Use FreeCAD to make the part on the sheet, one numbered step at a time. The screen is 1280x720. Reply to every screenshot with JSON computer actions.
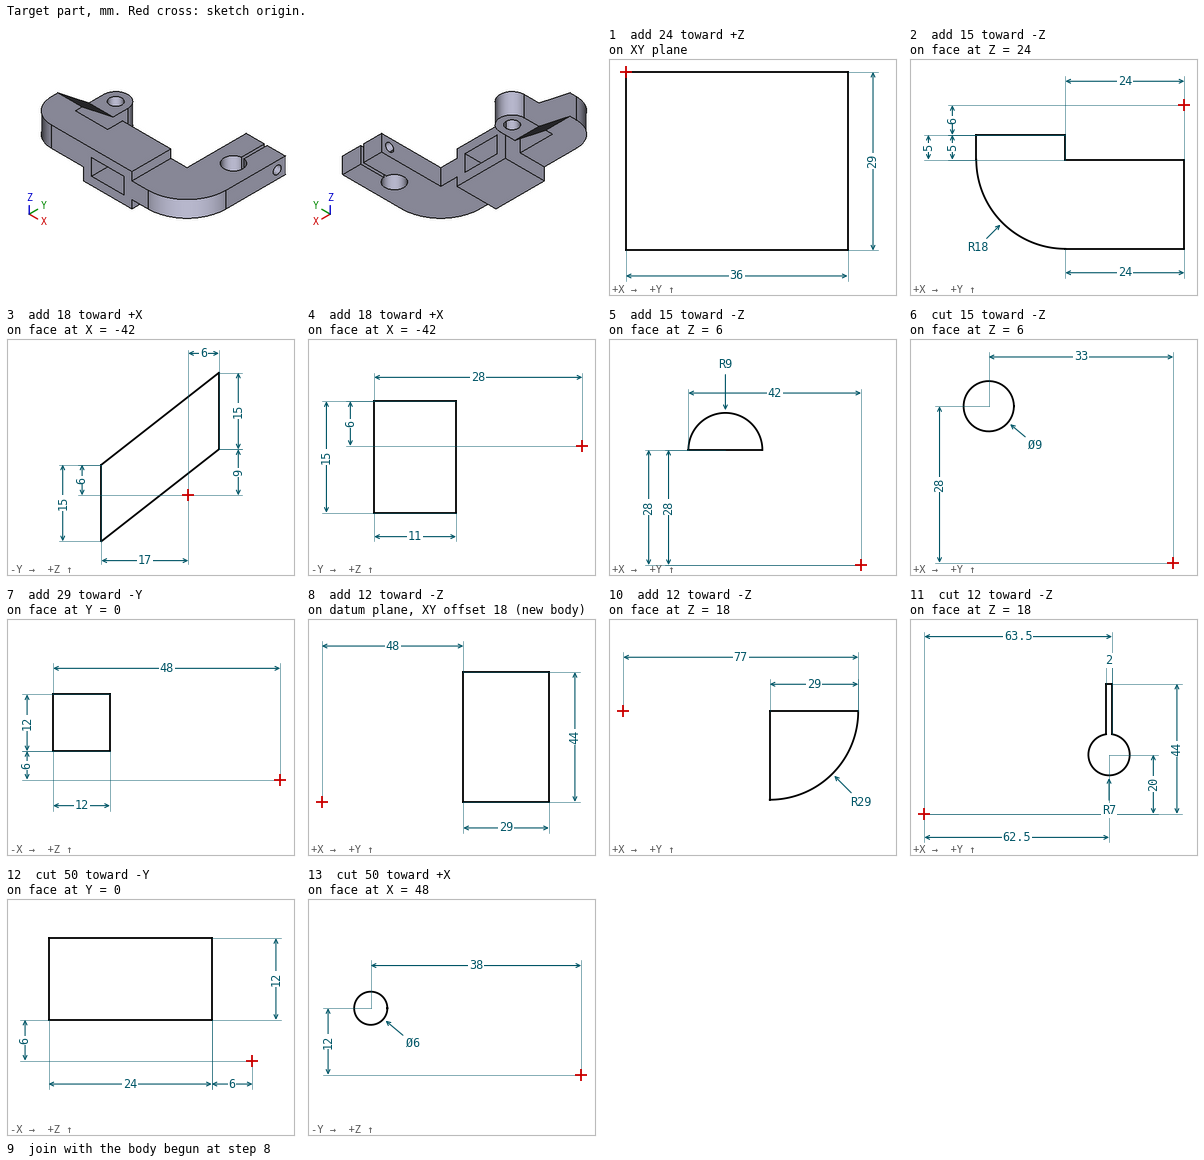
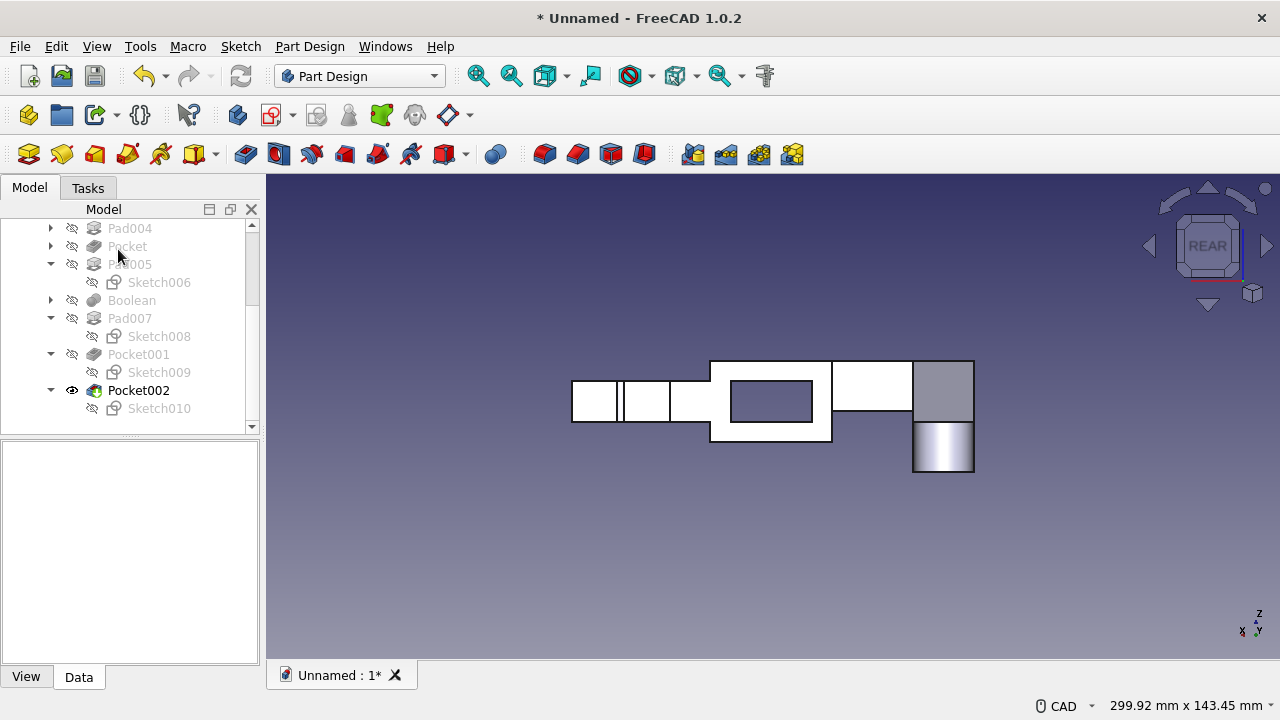
{"action": "left_click", "coordinate": [479, 76]}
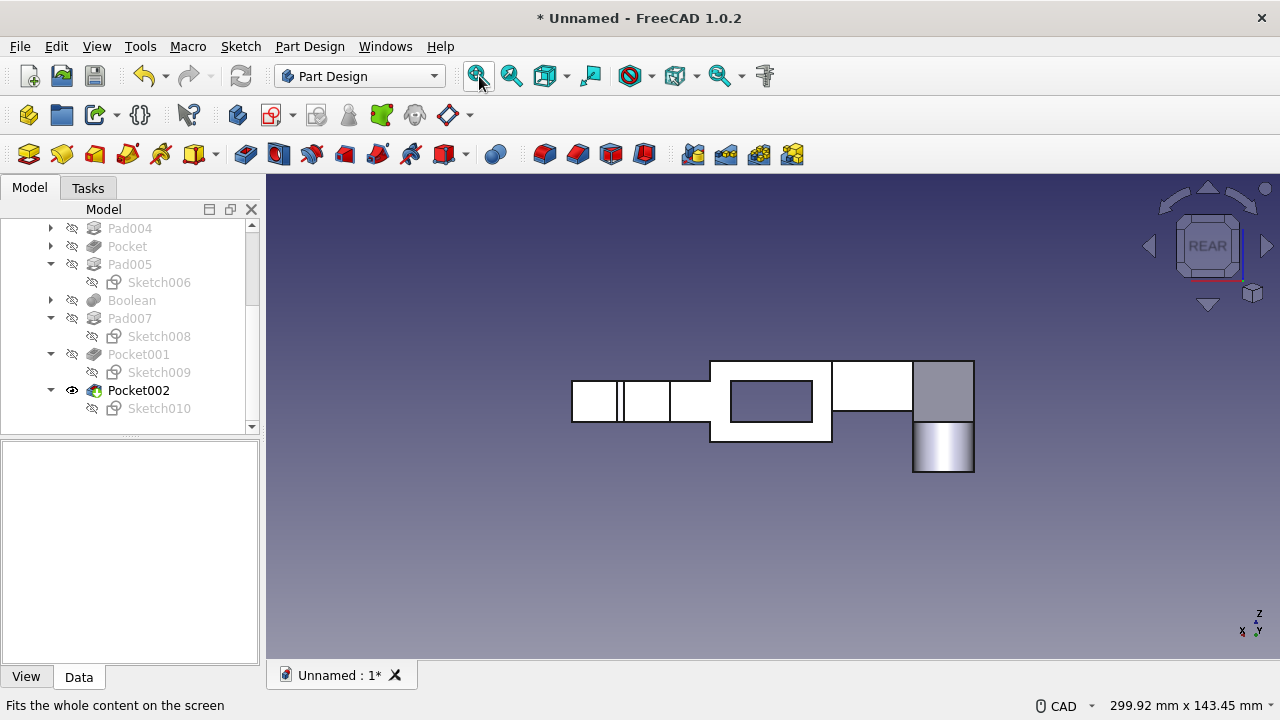
{"action": "key", "text": "6"}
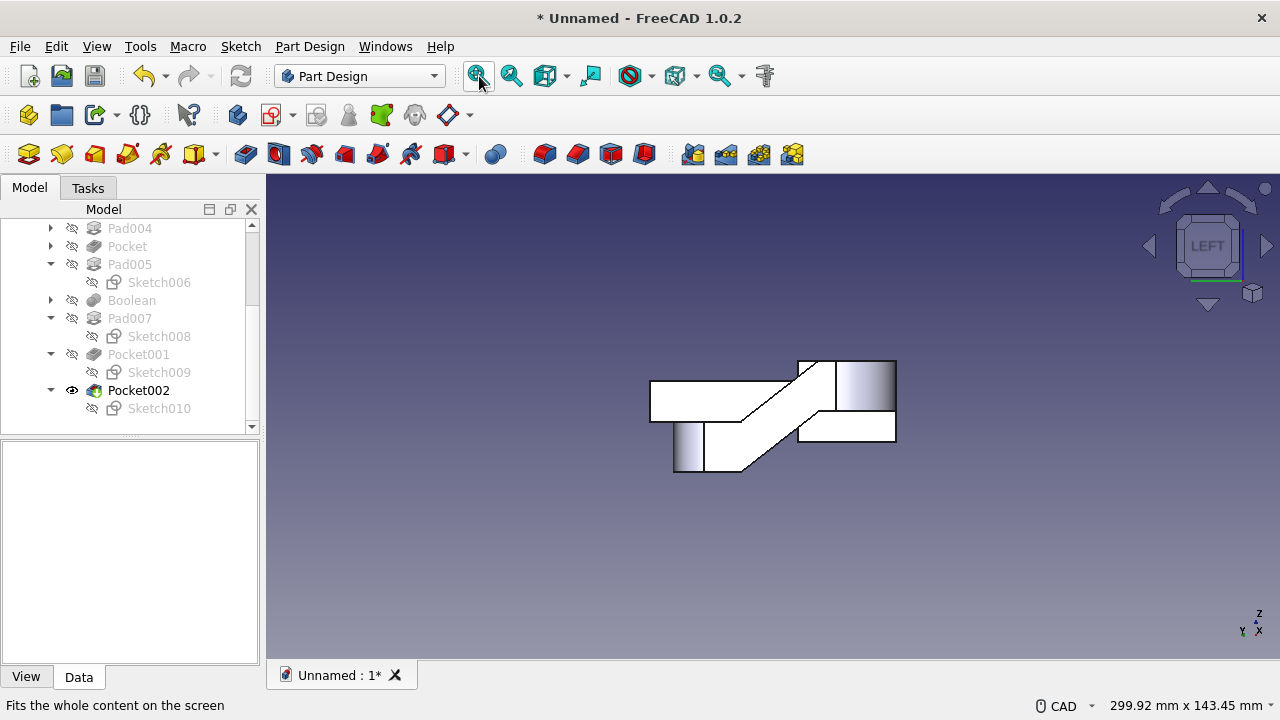
{"action": "left_click", "coordinate": [479, 76]}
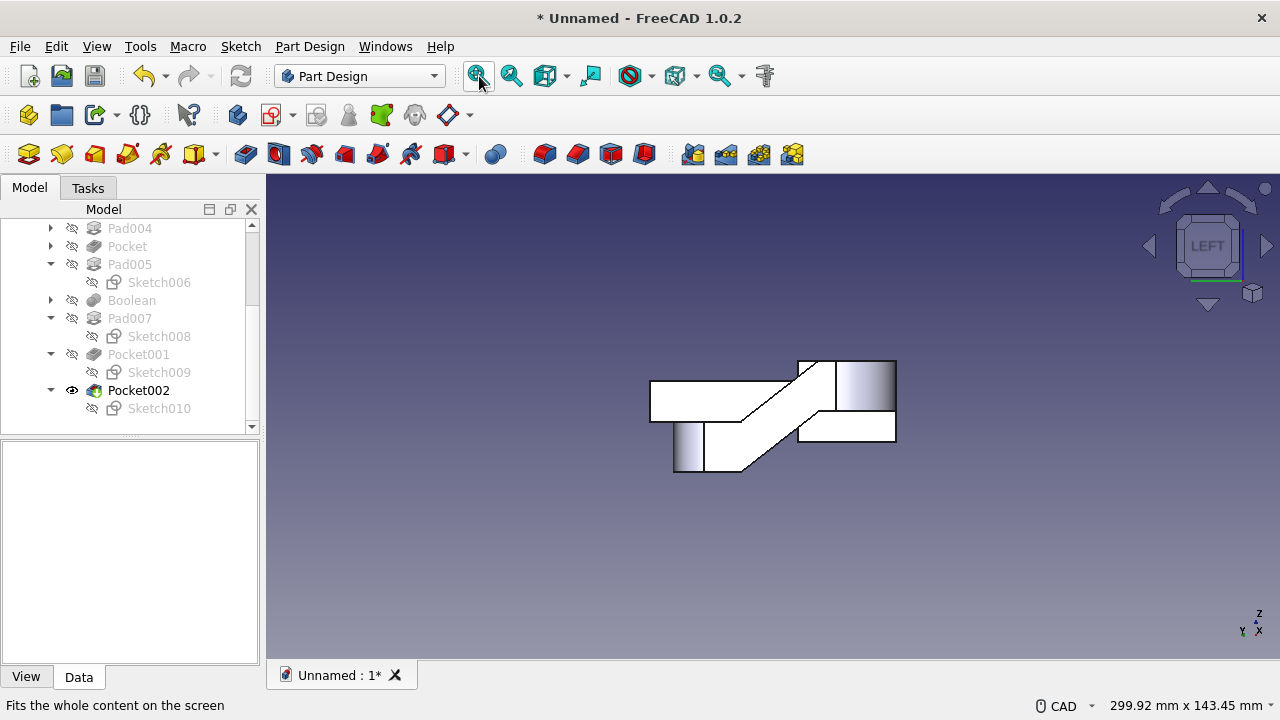
{"action": "left_click", "coordinate": [681, 400]}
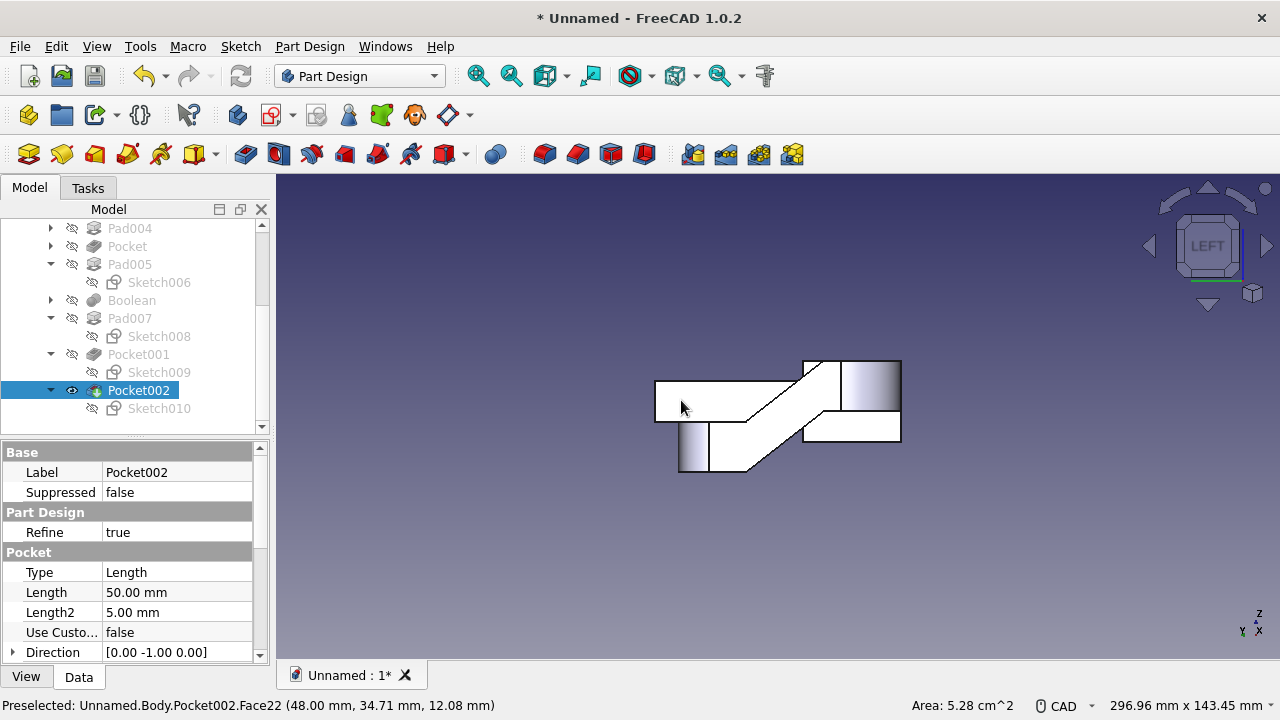
{"action": "left_click", "coordinate": [270, 116]}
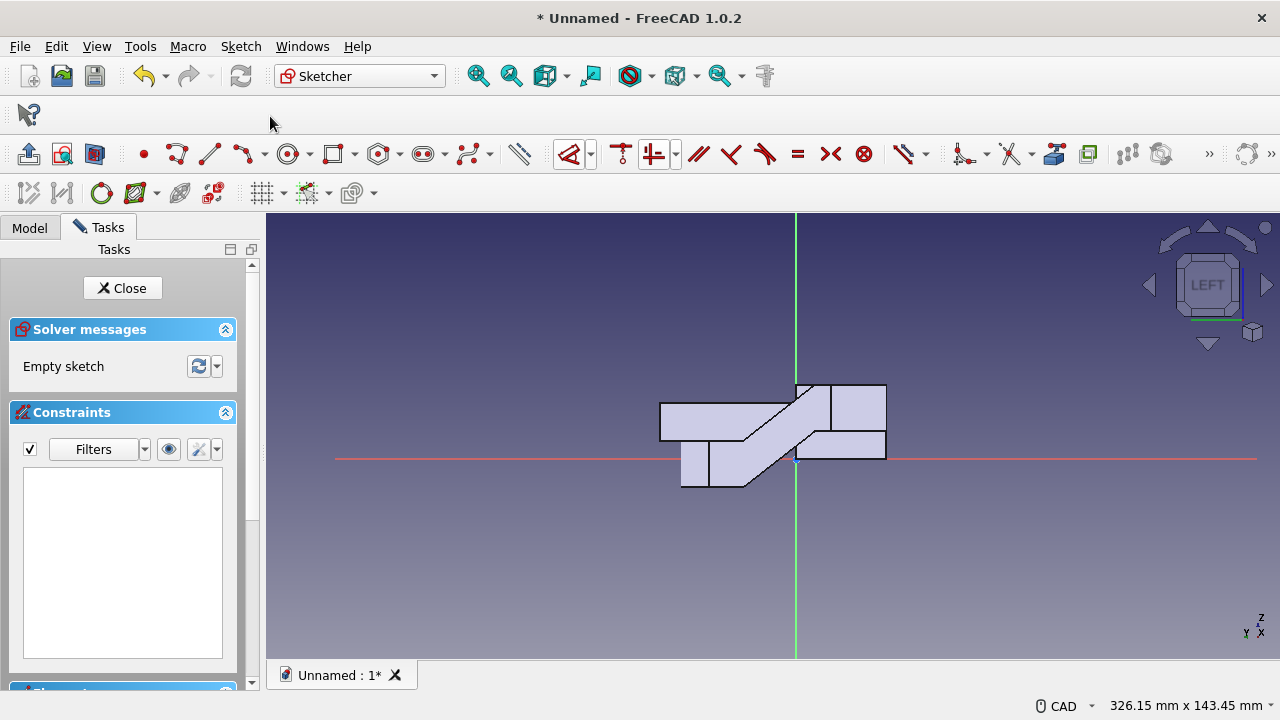
{"action": "scroll", "coordinate": [676, 421], "scroll_direction": "up", "scroll_amount": 13}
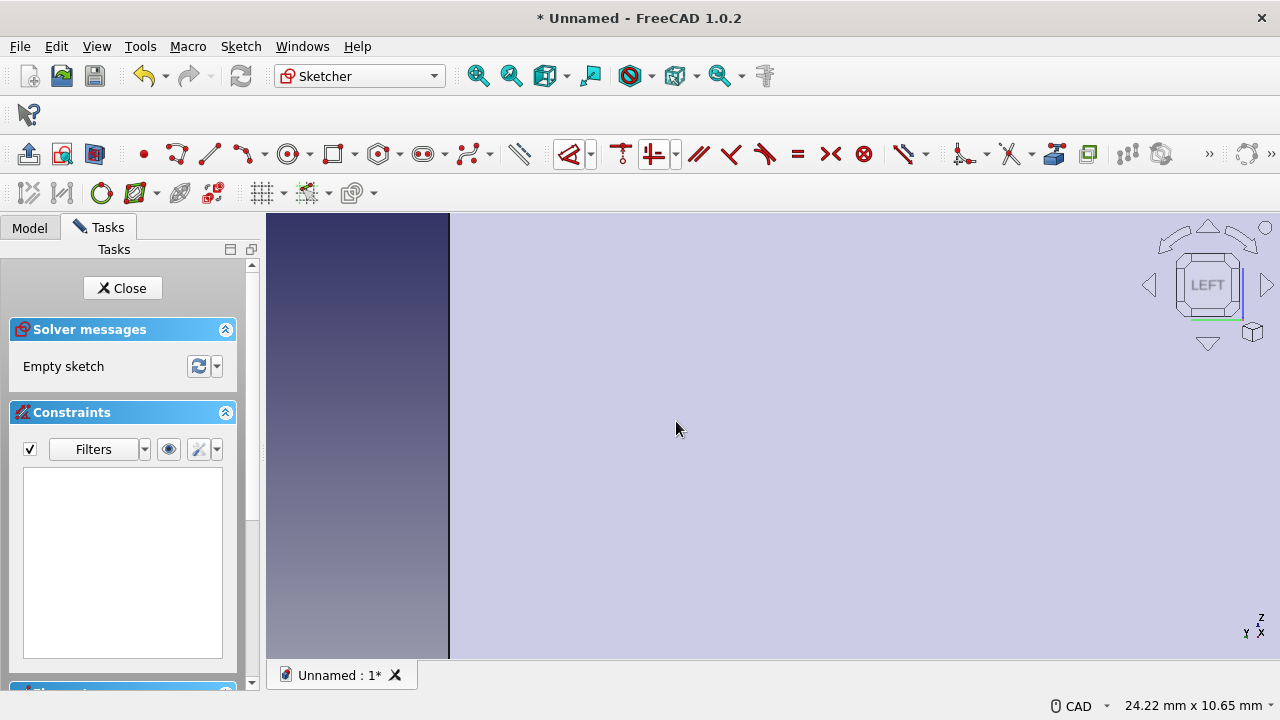
{"action": "left_click", "coordinate": [288, 154]}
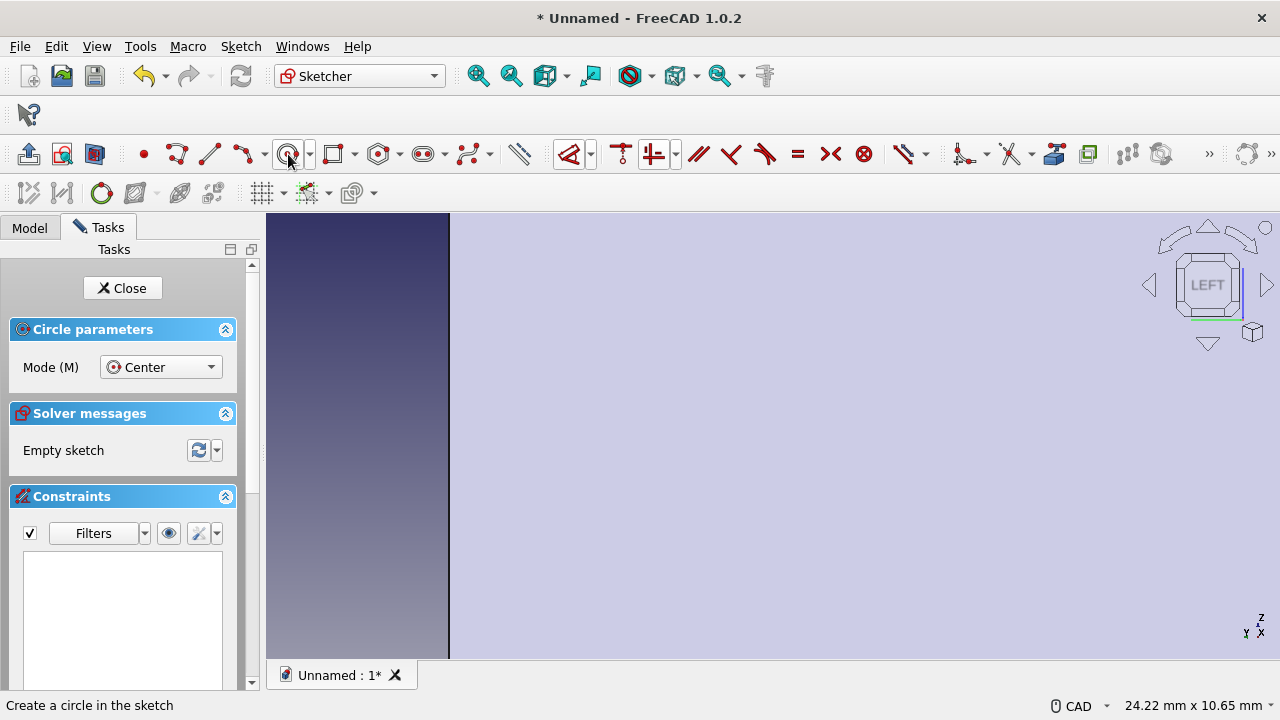
{"action": "left_click", "coordinate": [700, 429]}
{"action": "mouse_move", "coordinate": [789, 340]}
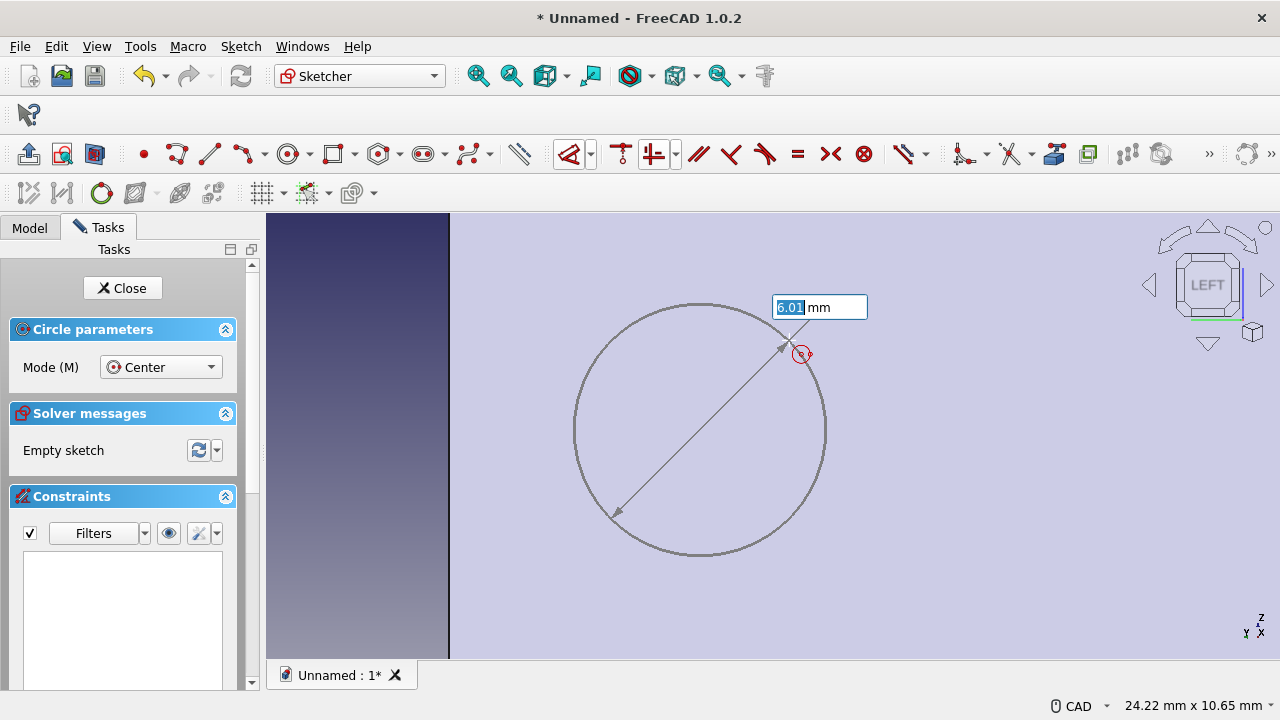
{"action": "type", "text": "6"}
{"action": "key", "text": "Return"}
{"action": "key", "text": "Escape"}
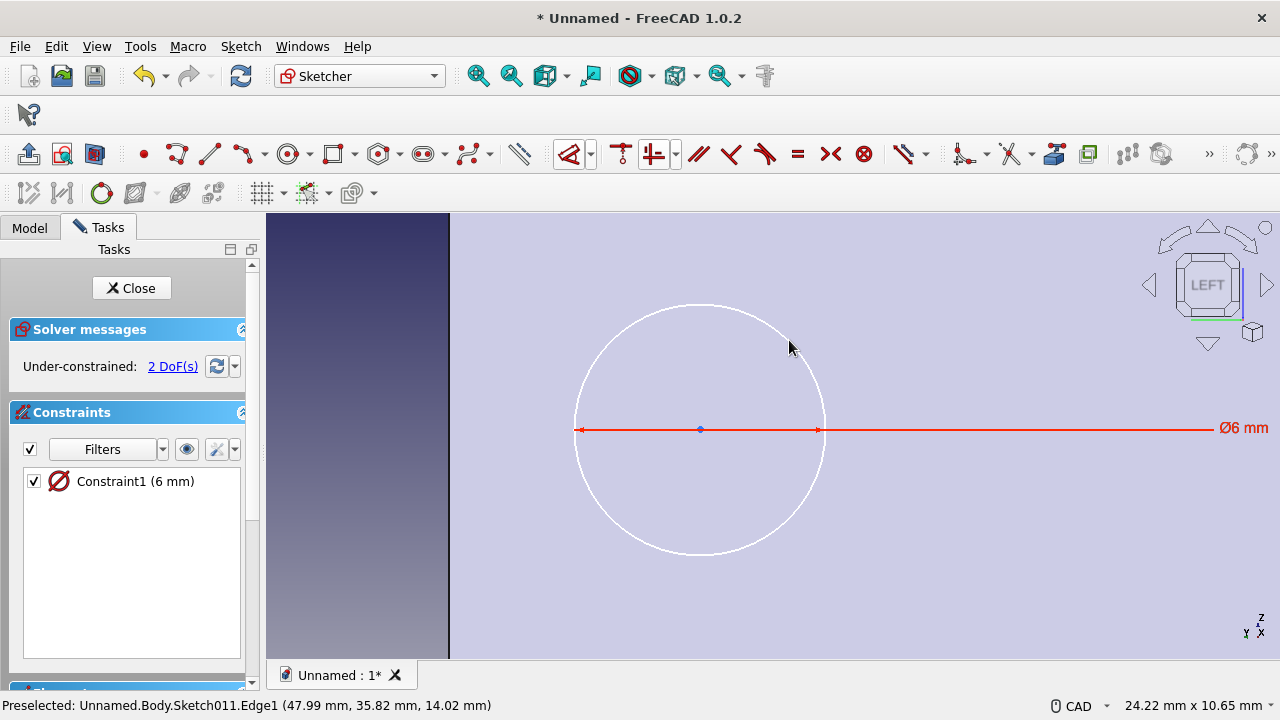
{"action": "left_click", "coordinate": [700, 430]}